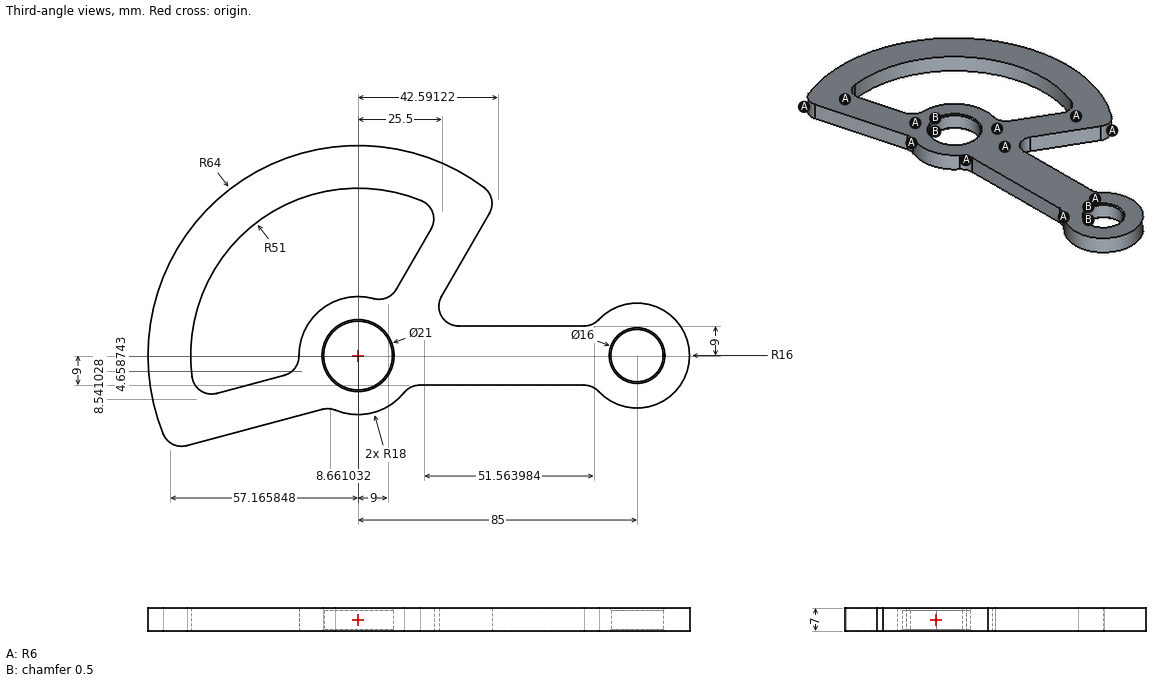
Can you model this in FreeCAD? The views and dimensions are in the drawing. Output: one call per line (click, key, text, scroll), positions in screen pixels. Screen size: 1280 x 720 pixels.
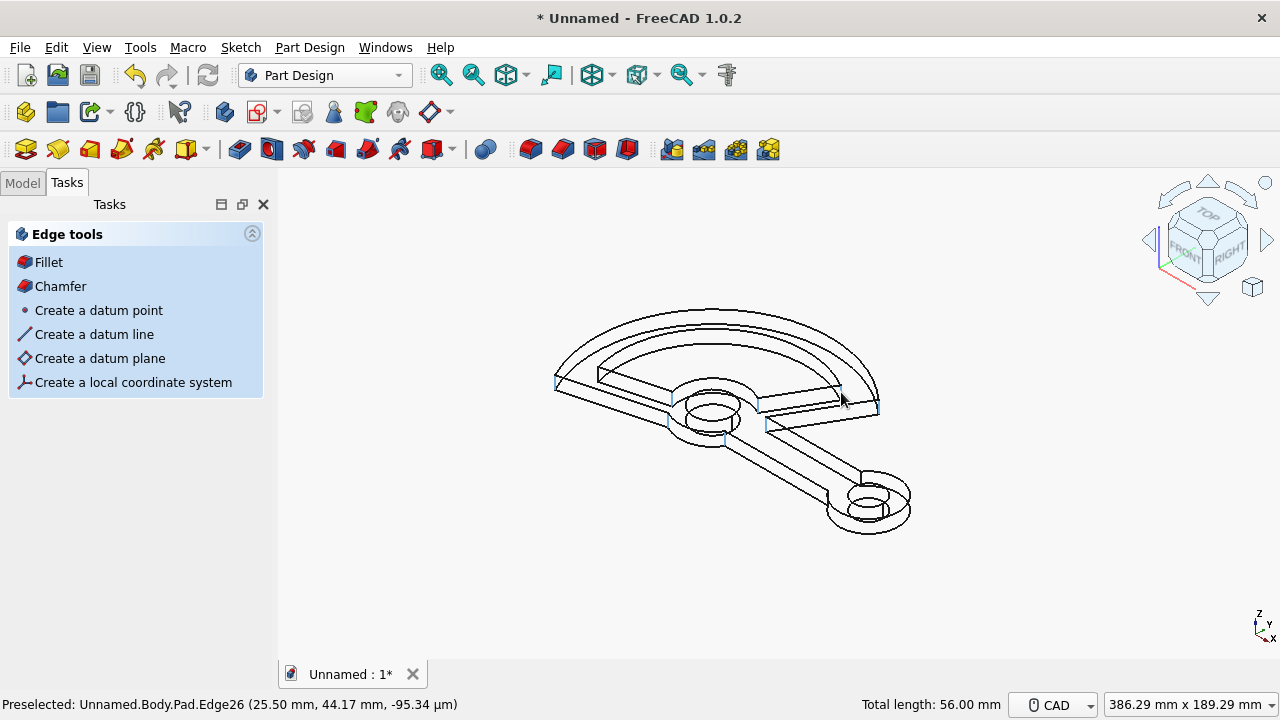
click(598, 373, ctrl)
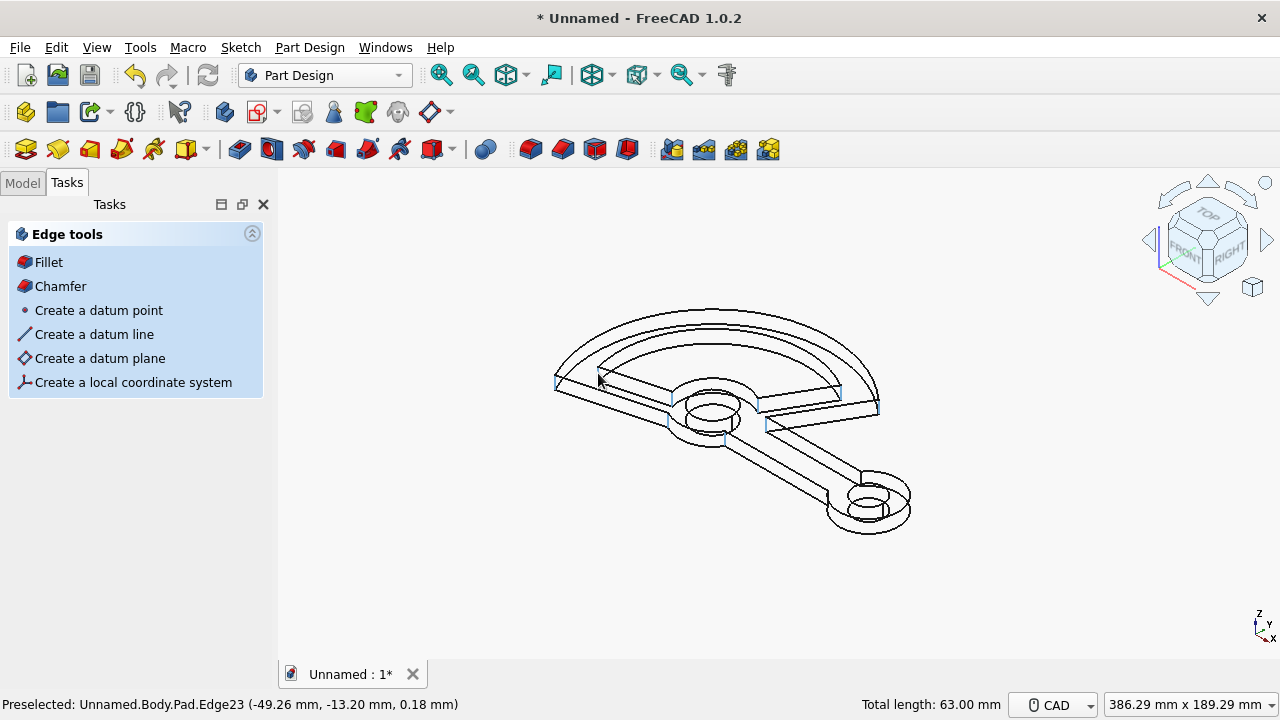
scroll(828, 497, up, 6)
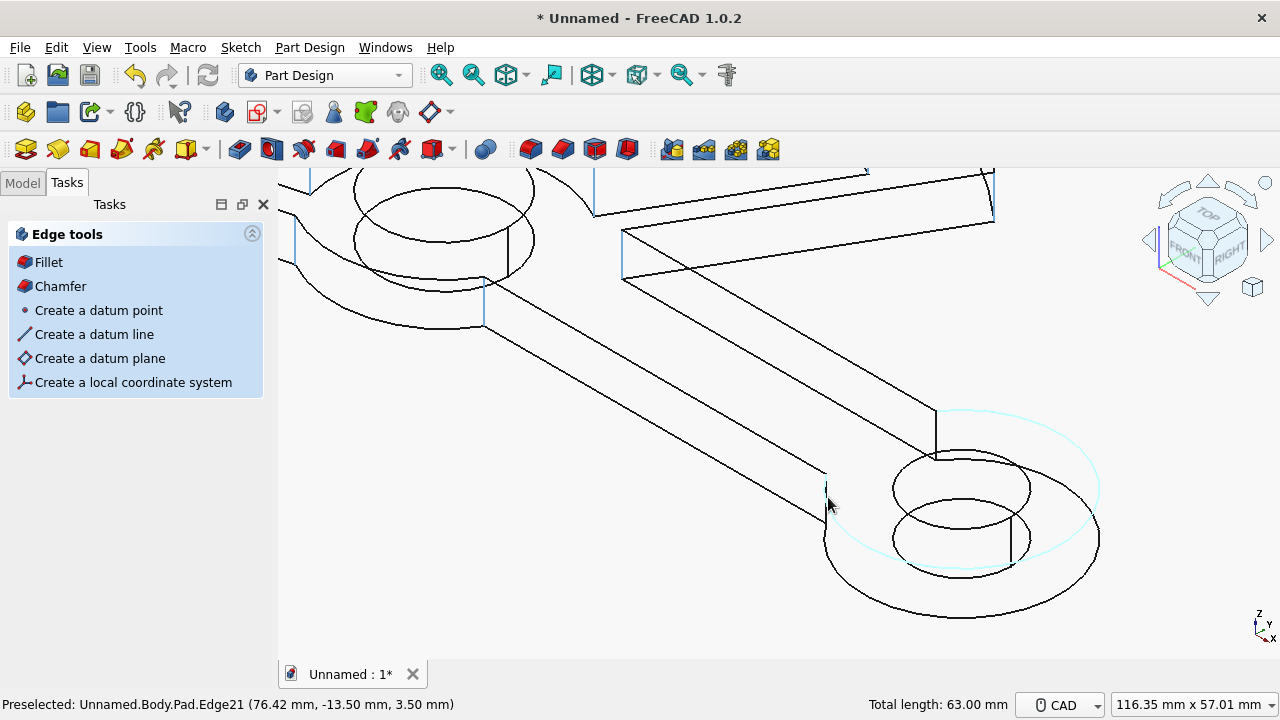
click(826, 517, ctrl)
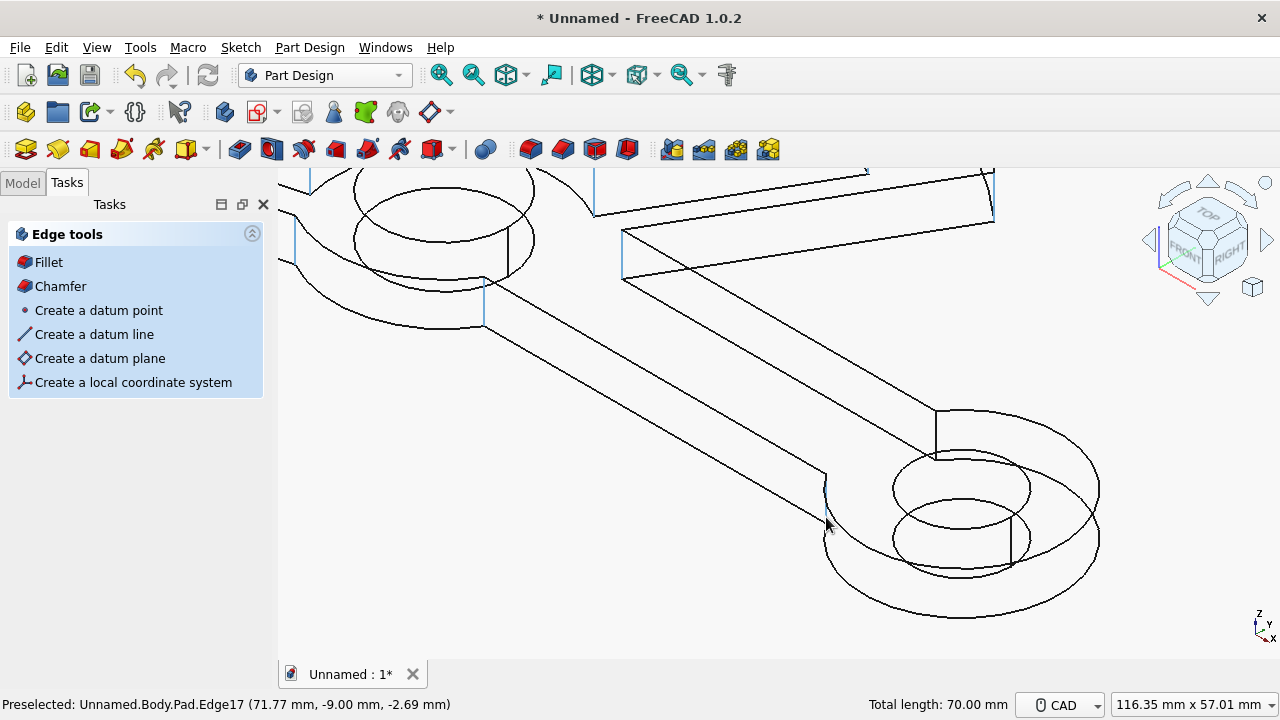
click(936, 435, ctrl)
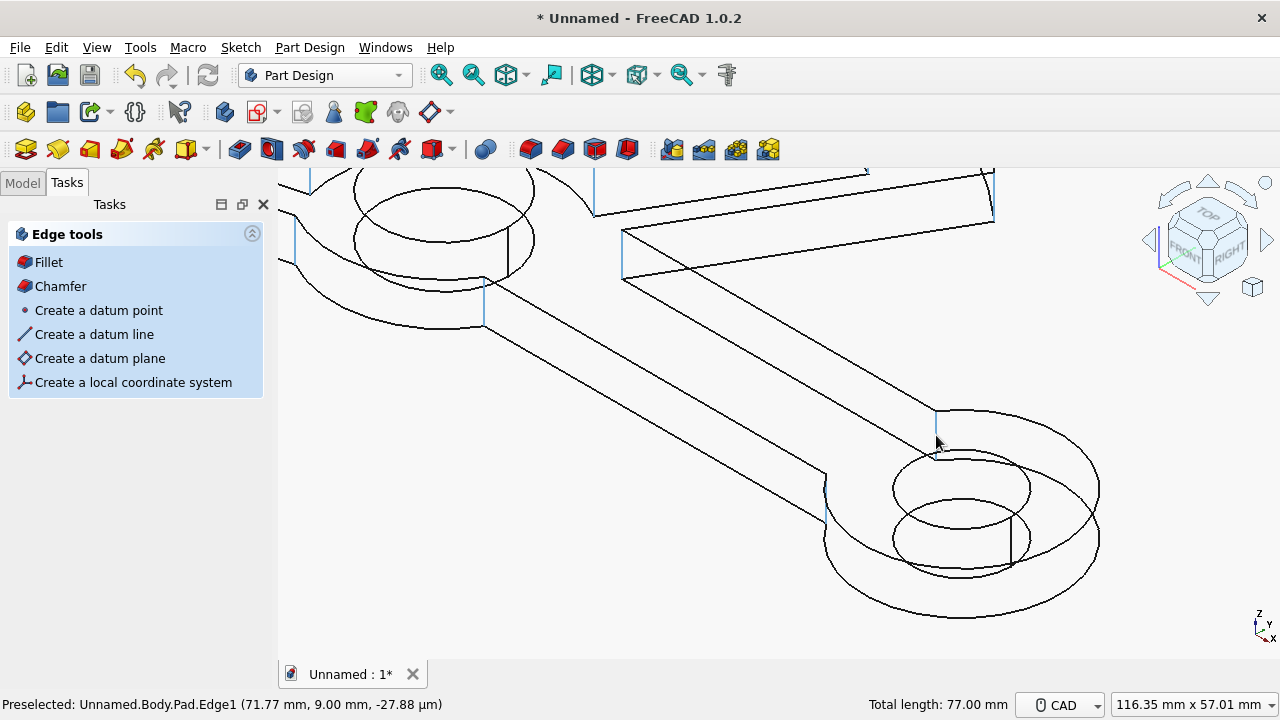
key(v)
key(1)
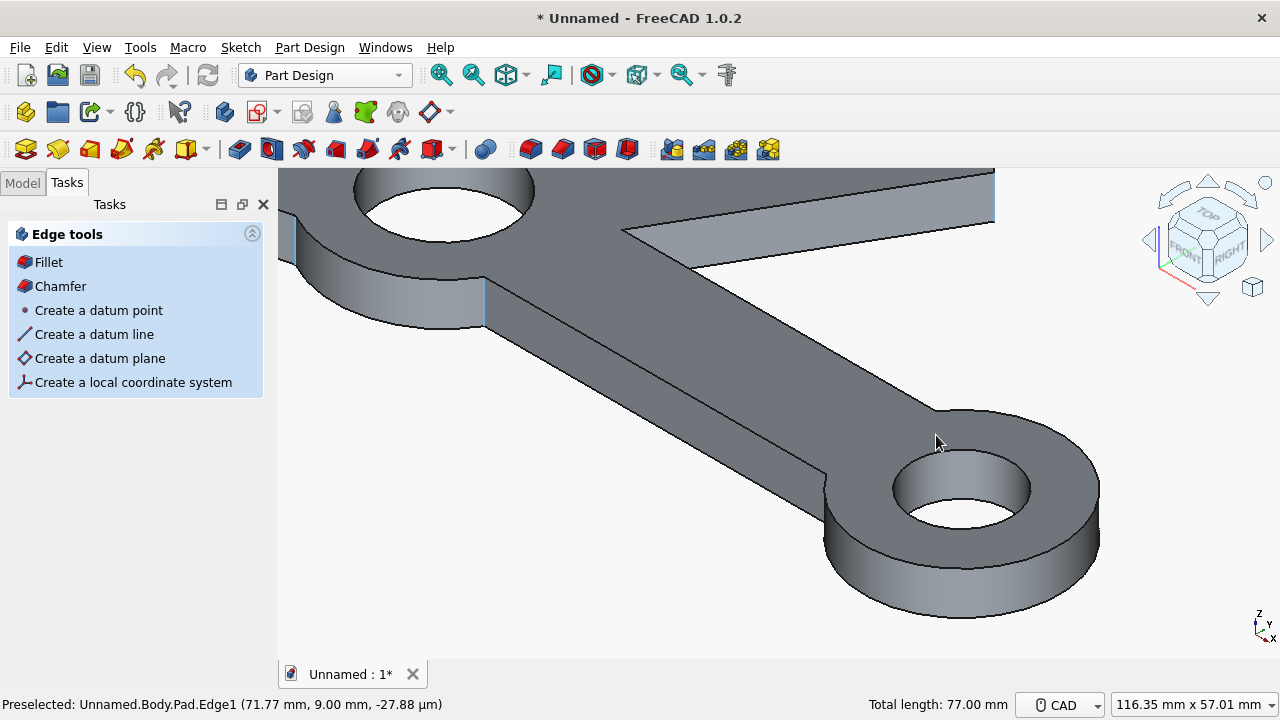
click(532, 150)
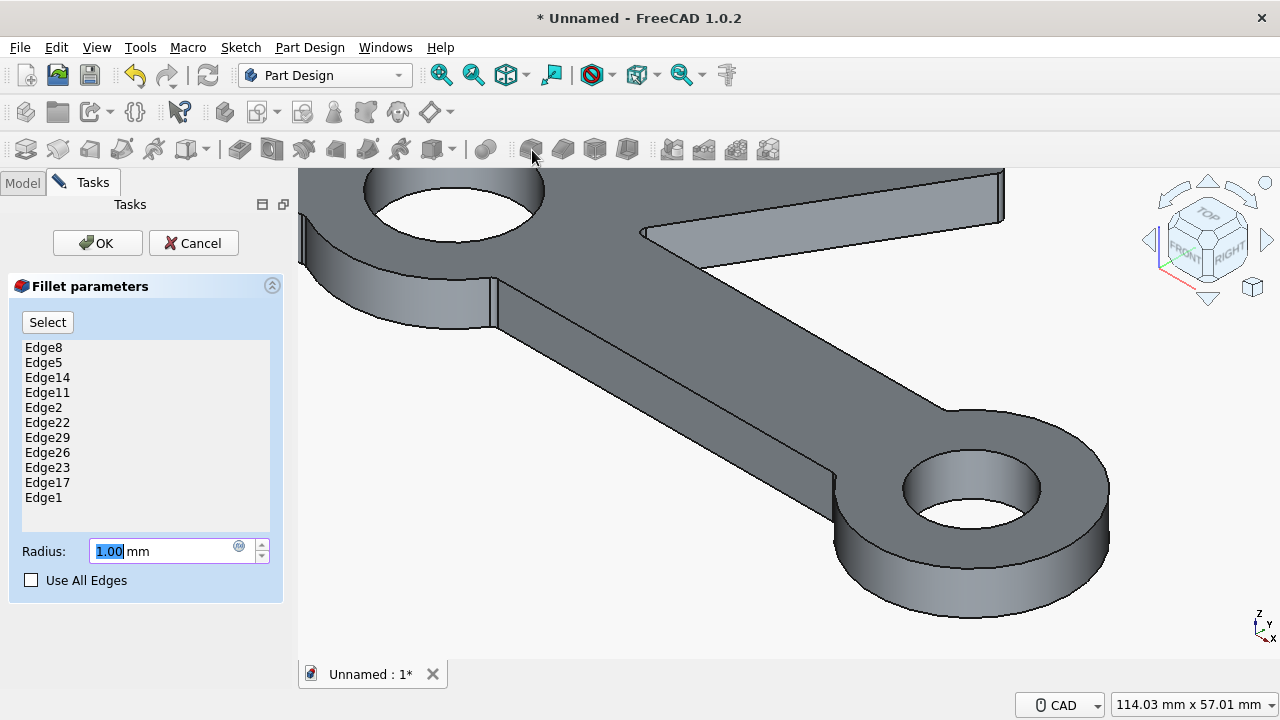
text(6)
key(Tab)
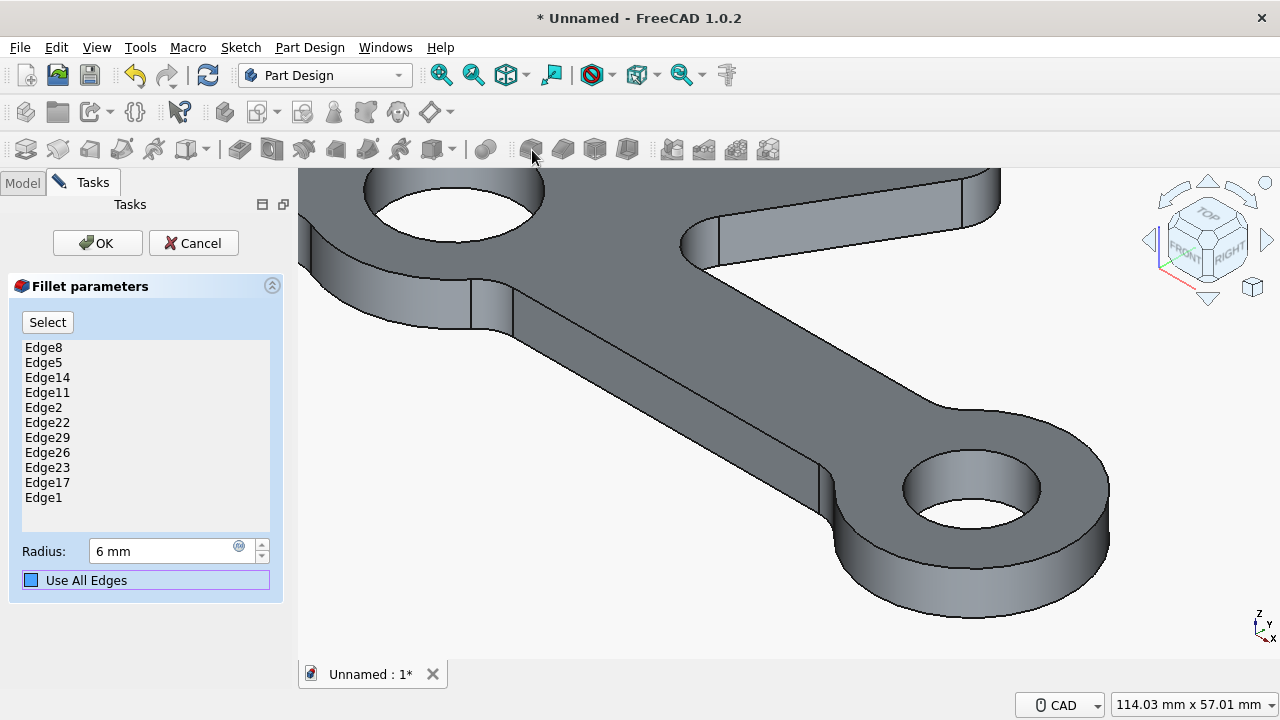
click(98, 243)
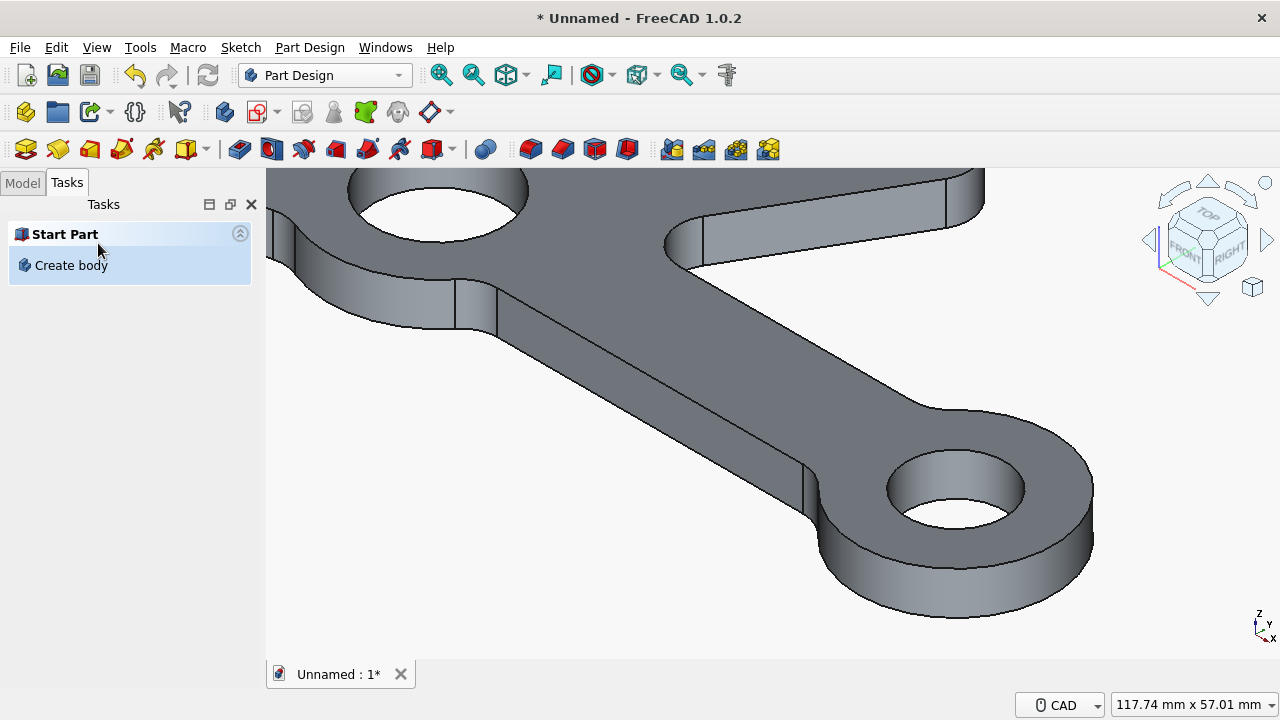
click(442, 76)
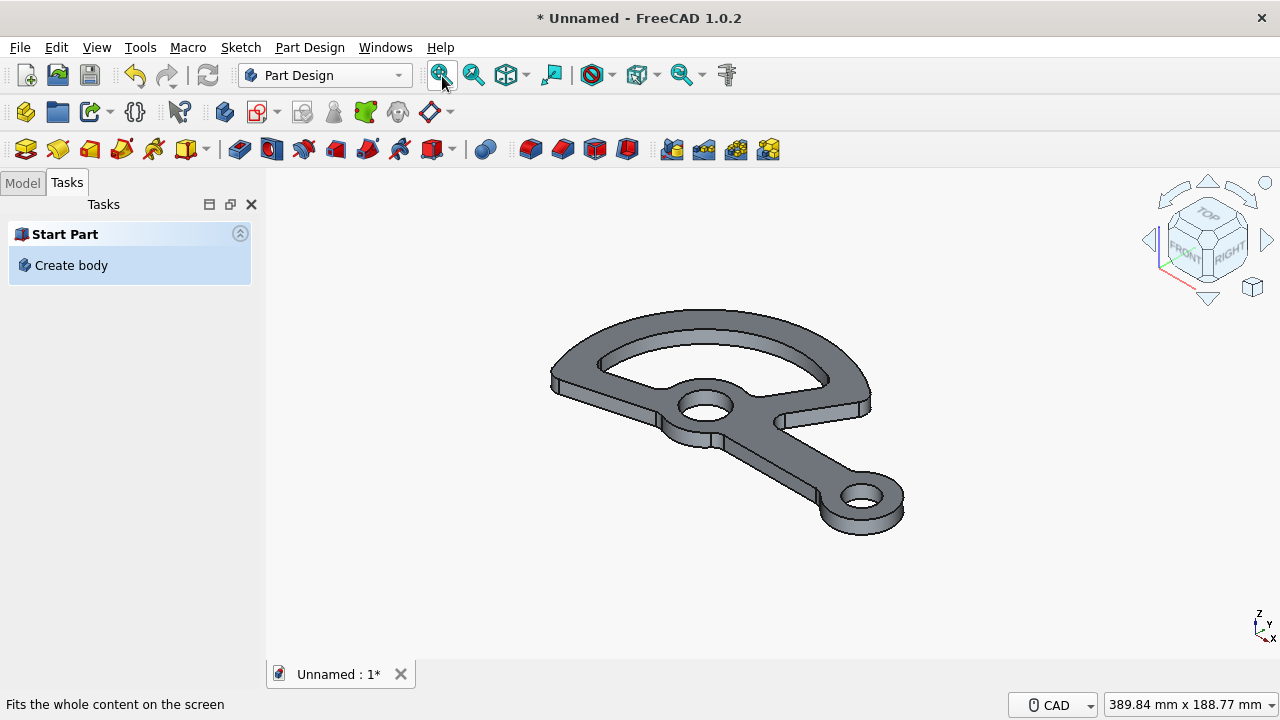
click(847, 487)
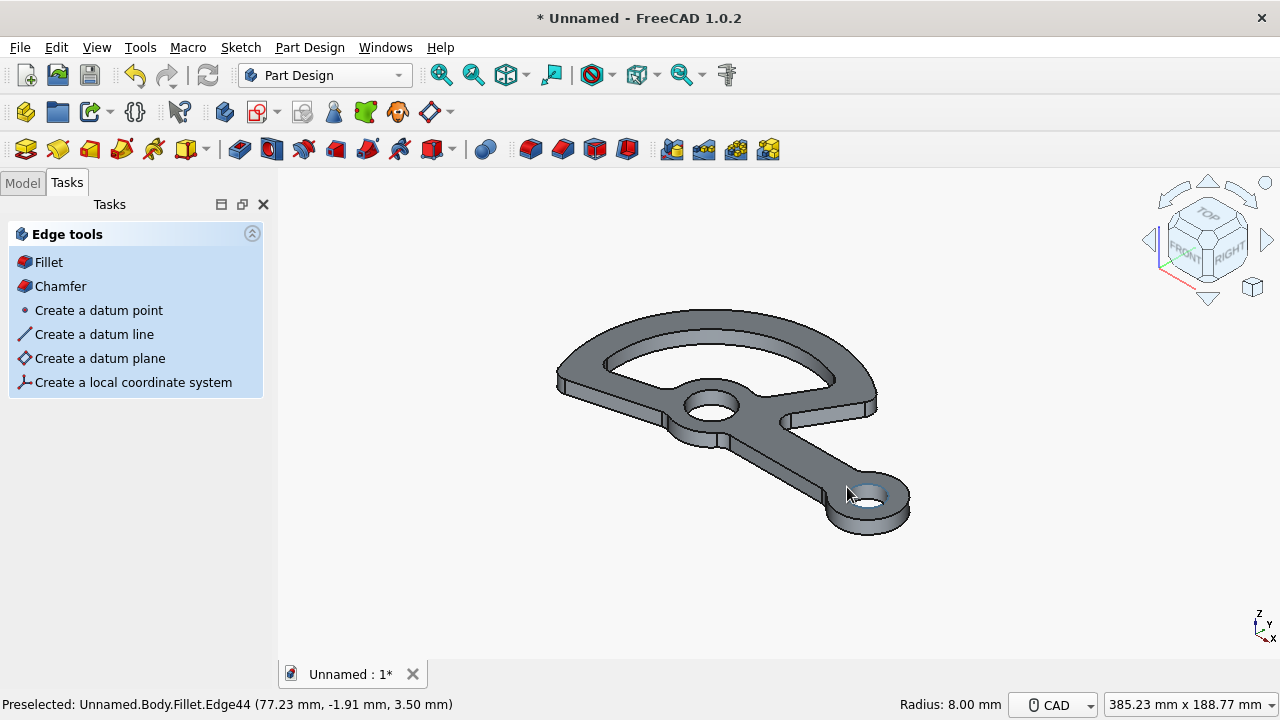
click(692, 394, ctrl)